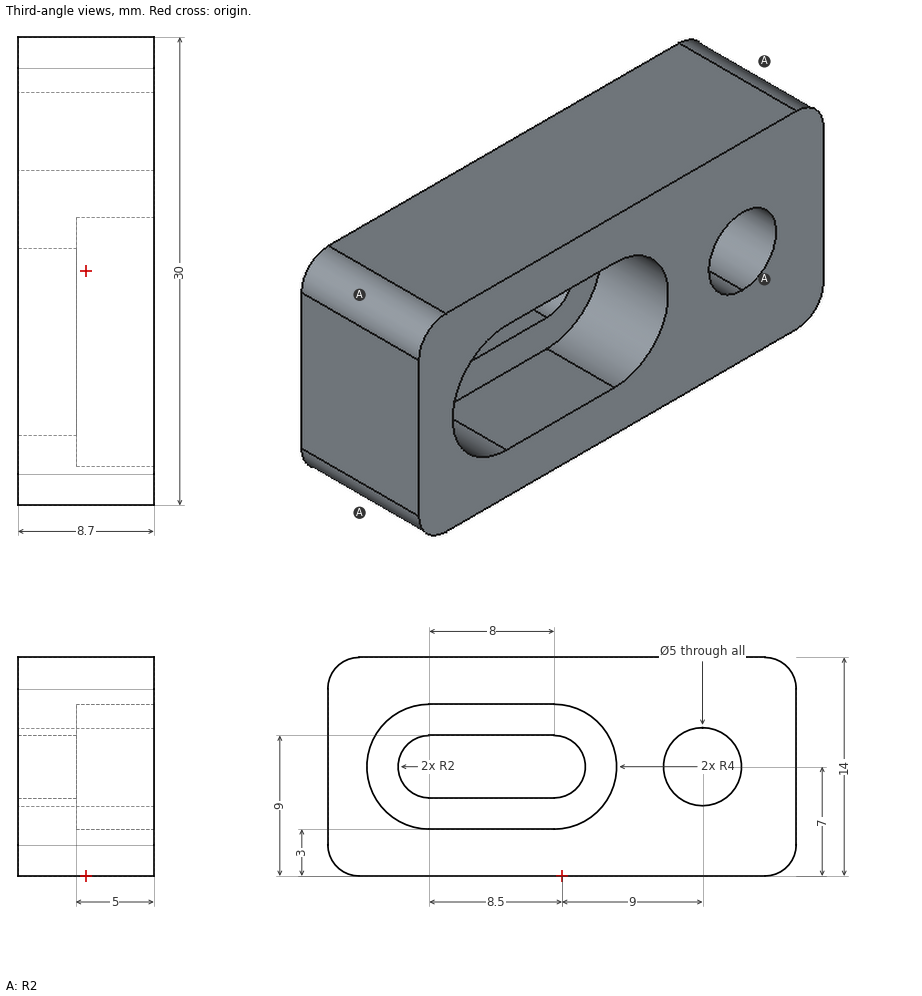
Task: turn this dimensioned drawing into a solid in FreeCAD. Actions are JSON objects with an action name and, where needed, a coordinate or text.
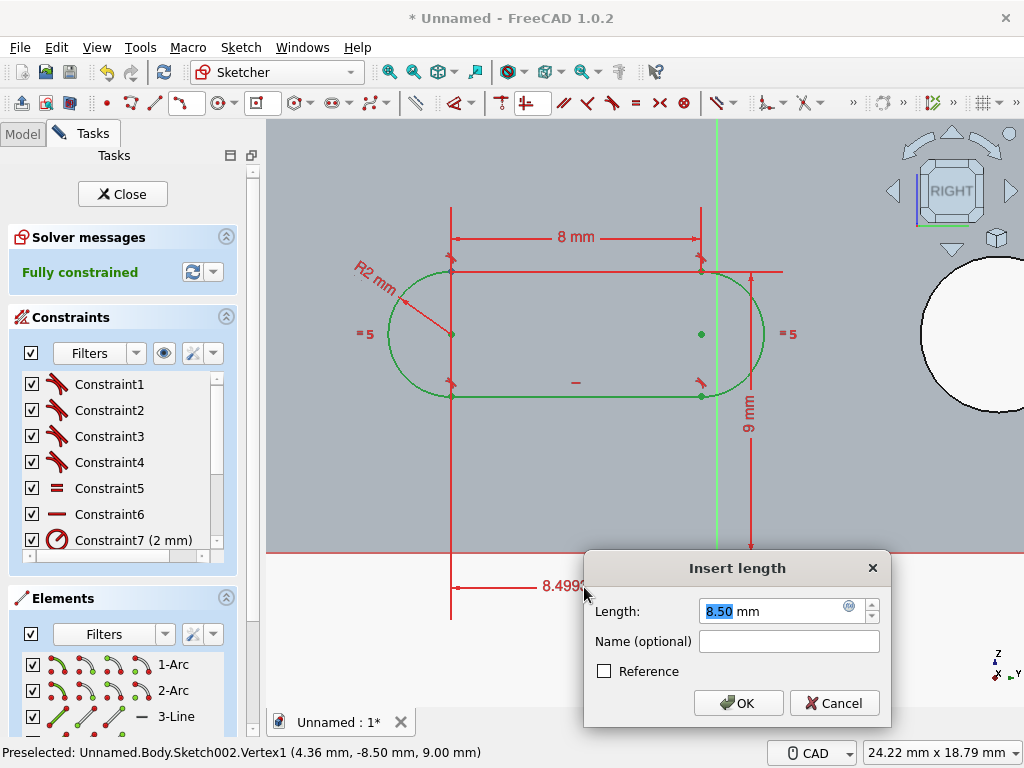
{"action": "type", "text": "8.5"}
{"action": "key", "text": "Return"}
{"action": "key", "text": "Escape"}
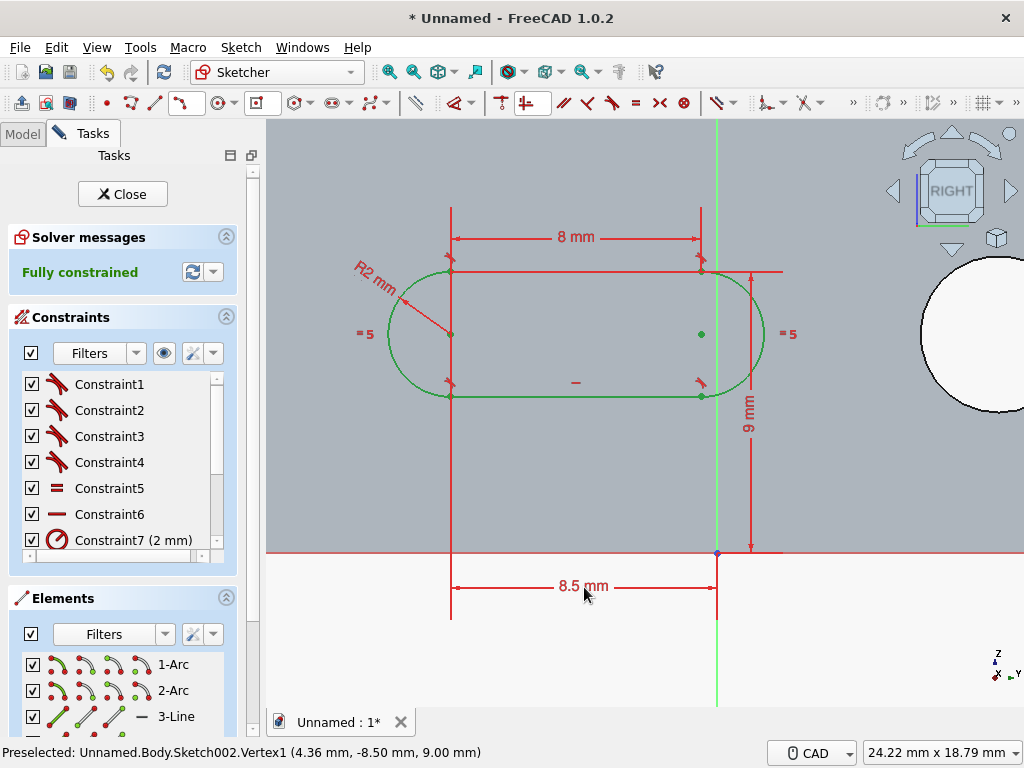
{"action": "left_click", "coordinate": [123, 194]}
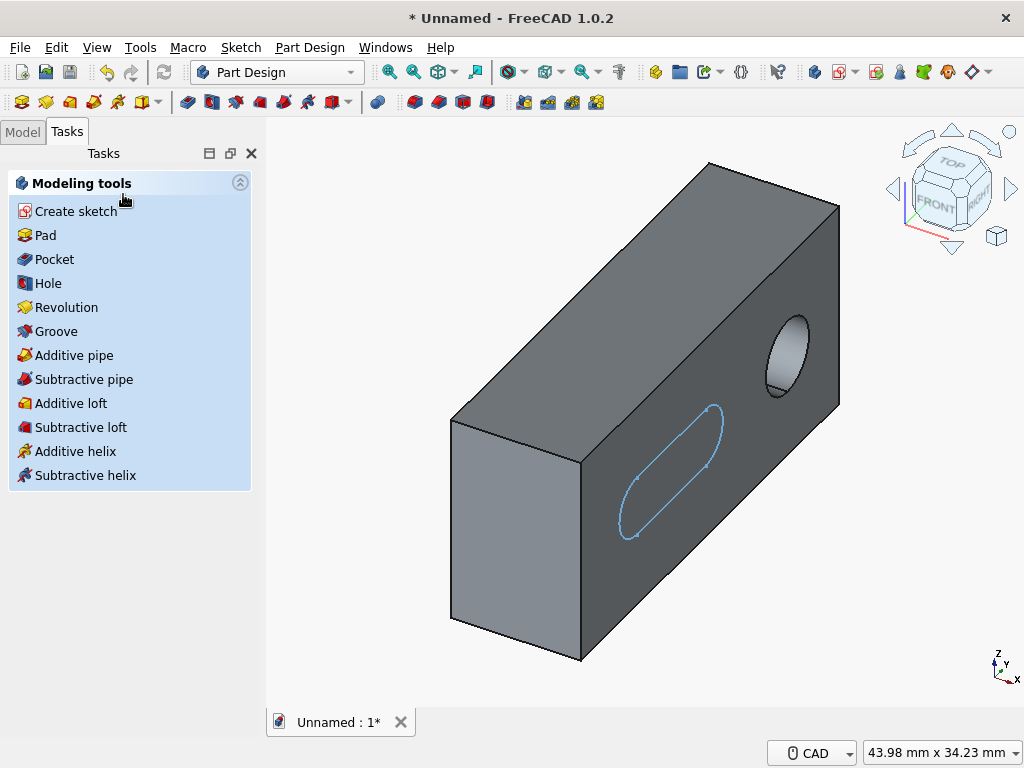
{"action": "left_click", "coordinate": [188, 102]}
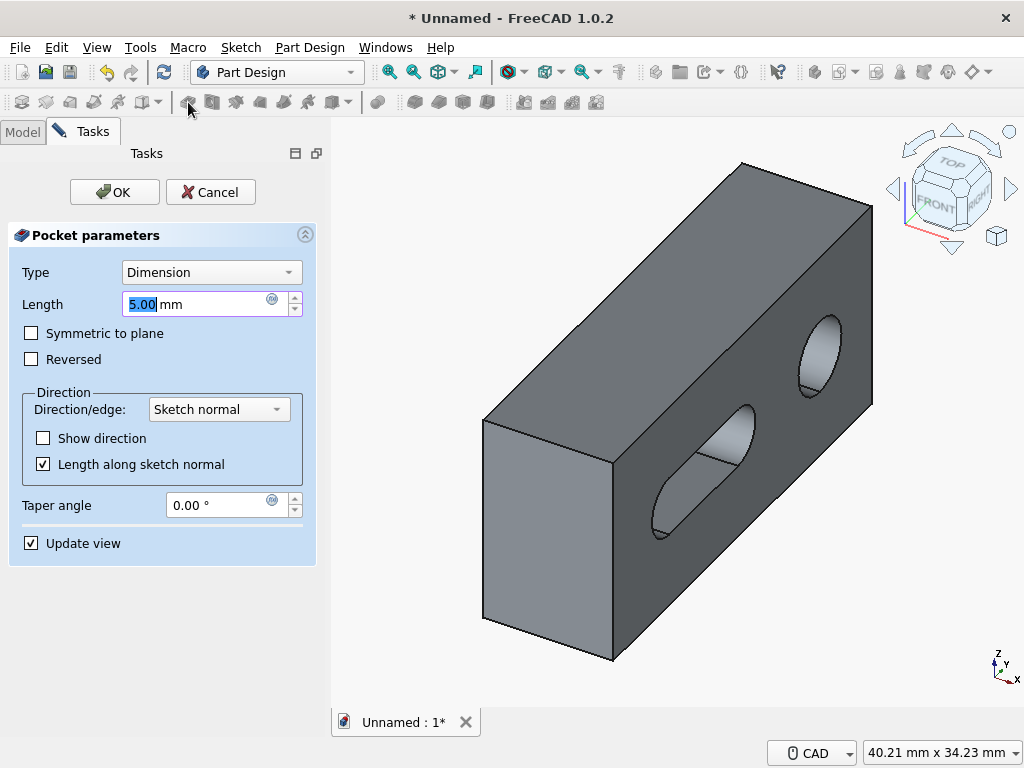
{"action": "left_click", "coordinate": [212, 272]}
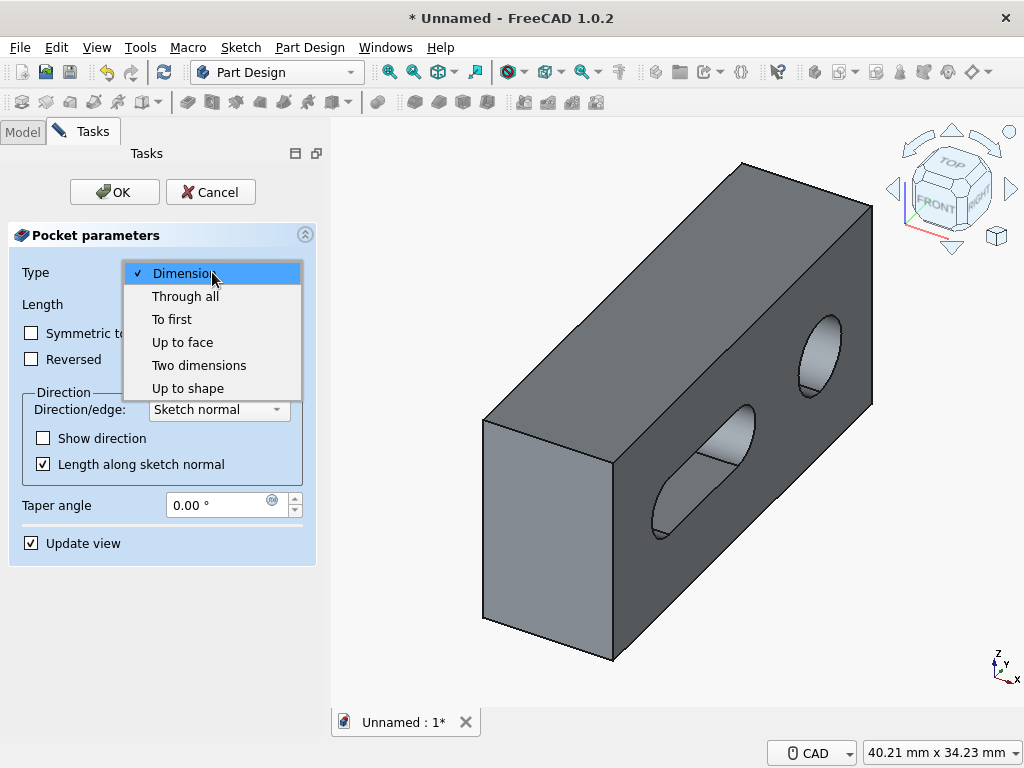
{"action": "left_click", "coordinate": [212, 296]}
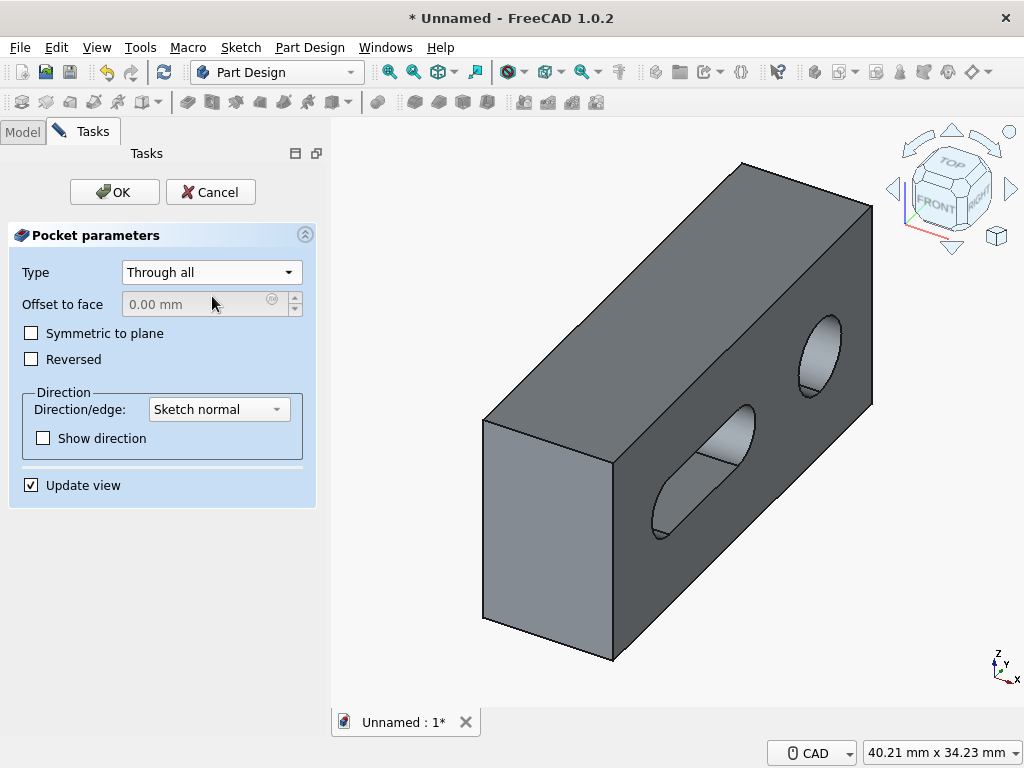
{"action": "left_click", "coordinate": [115, 192]}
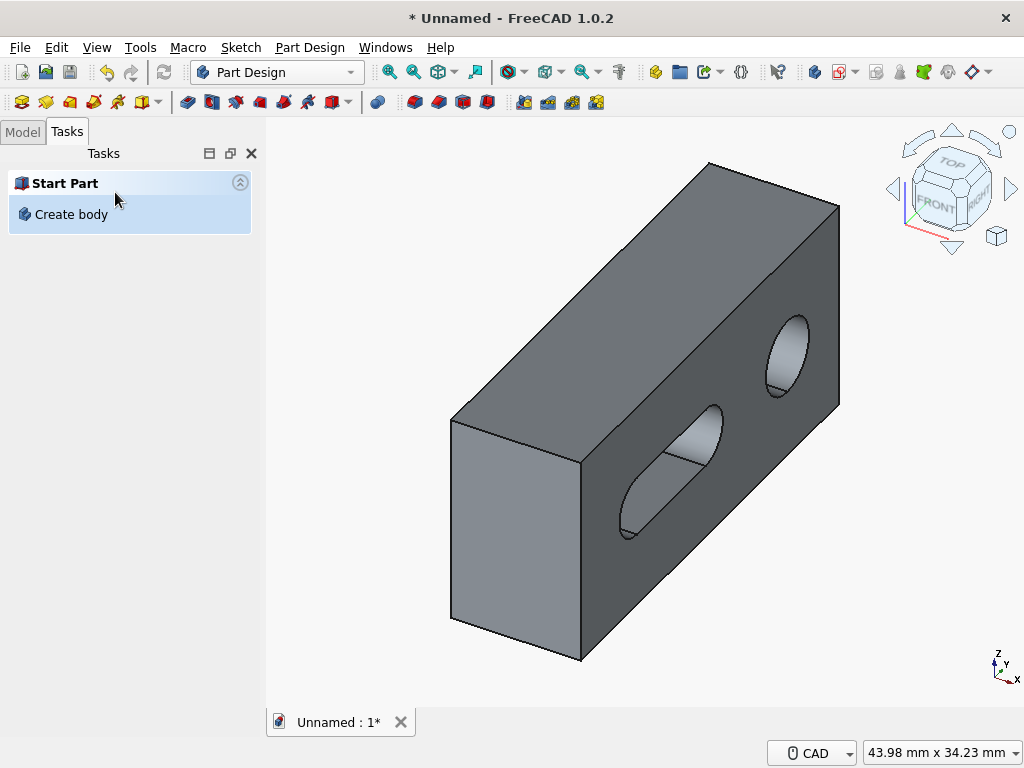
{"action": "left_click", "coordinate": [747, 339]}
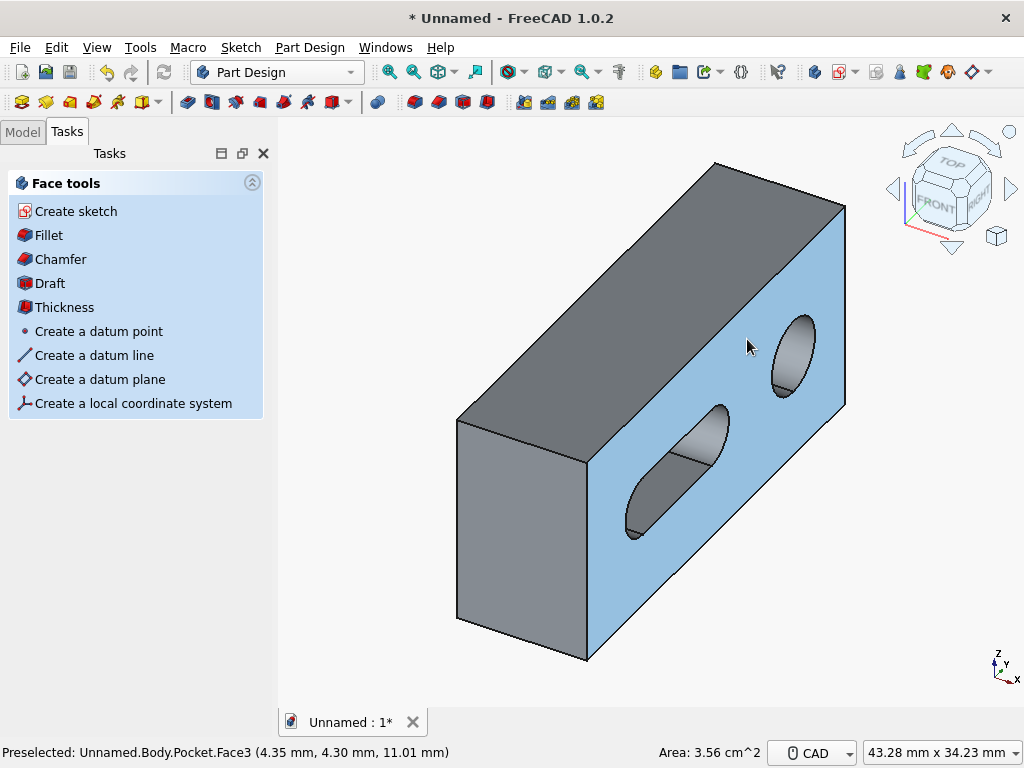
{"action": "left_click", "coordinate": [840, 72]}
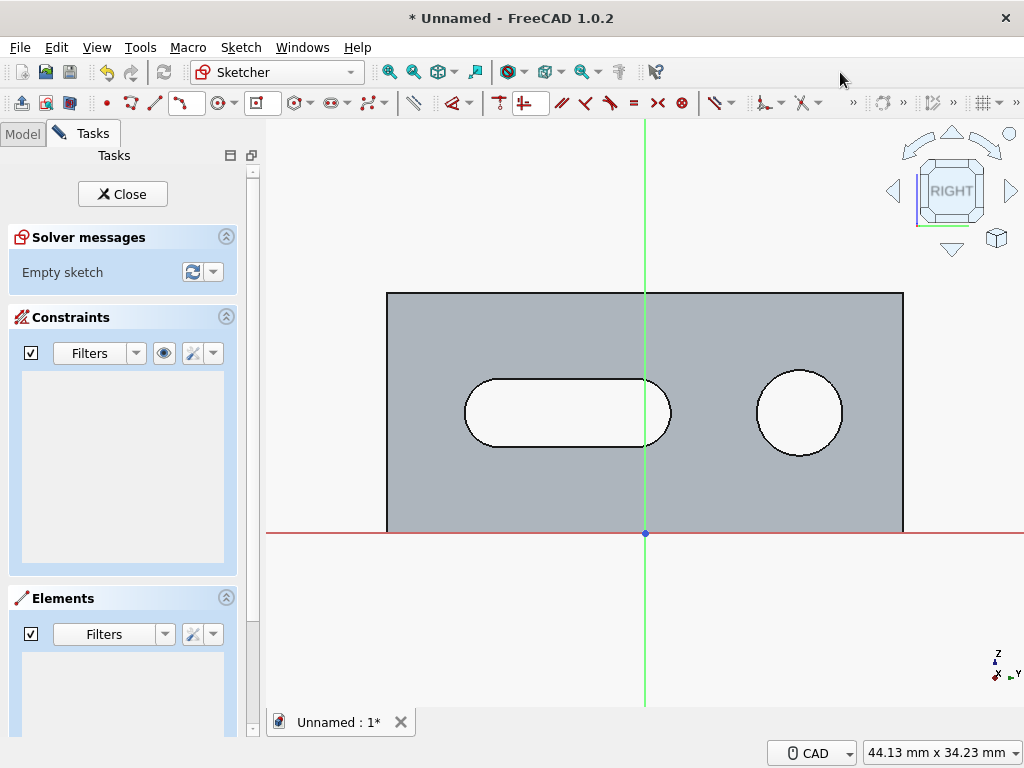
{"action": "scroll", "coordinate": [550, 491], "scroll_direction": "up", "scroll_amount": 2}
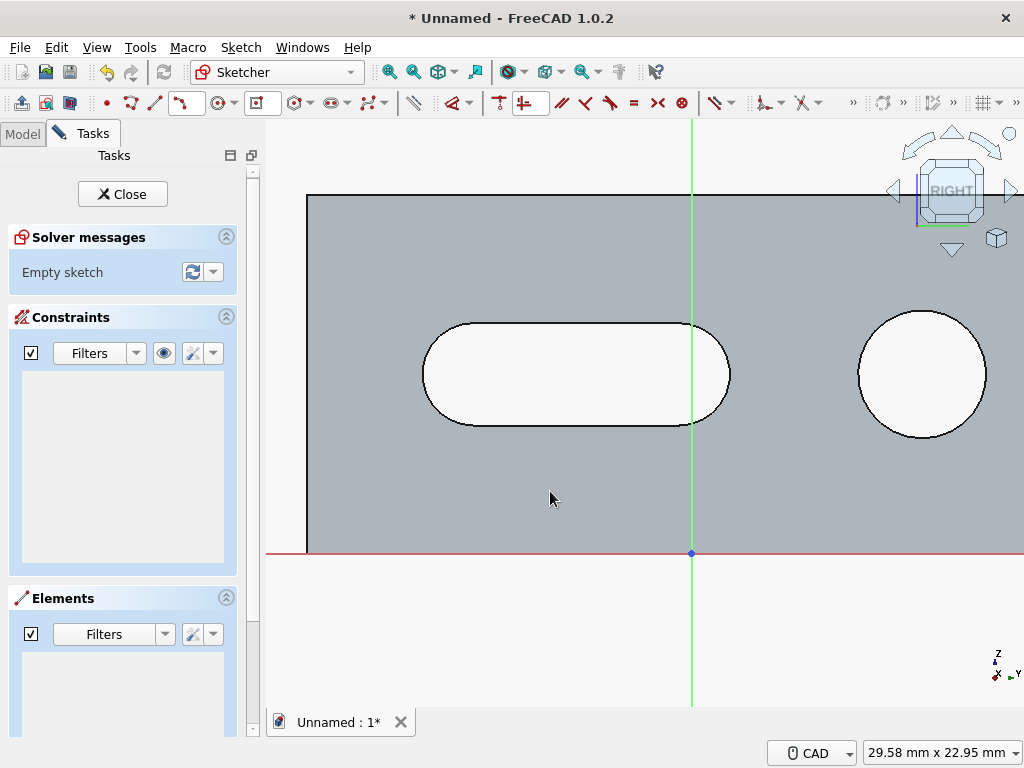
{"action": "left_click", "coordinate": [332, 104]}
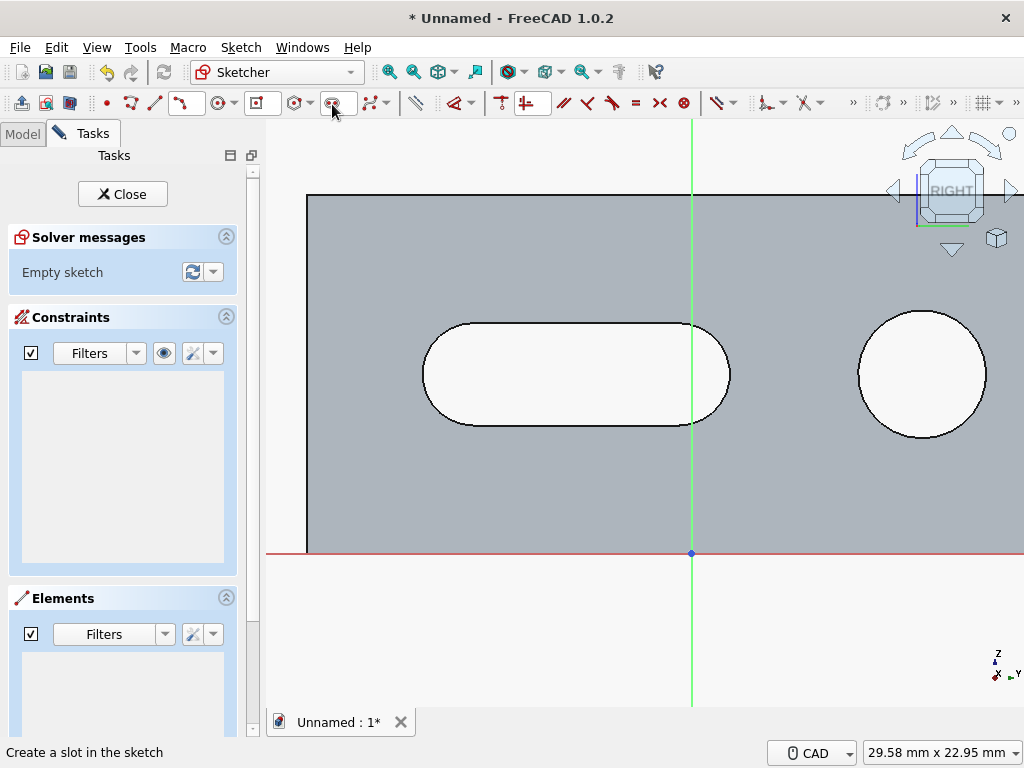
{"action": "left_click", "coordinate": [474, 374]}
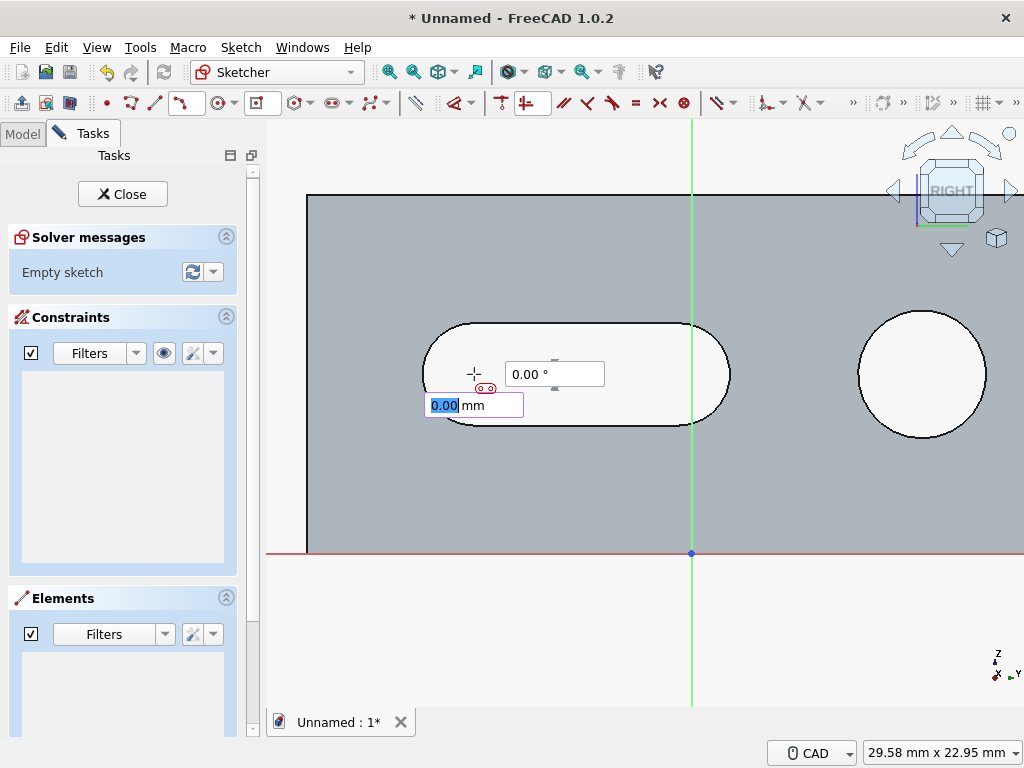
{"action": "scroll", "coordinate": [679, 374], "scroll_direction": "up", "scroll_amount": 2}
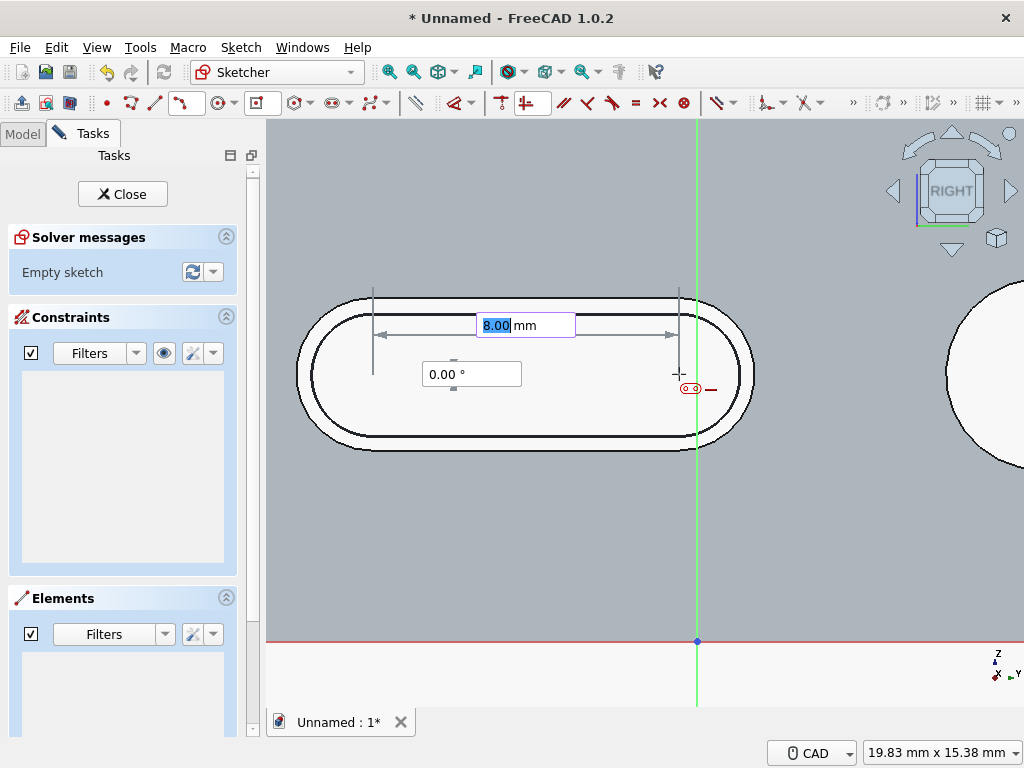
{"action": "left_click", "coordinate": [678, 374]}